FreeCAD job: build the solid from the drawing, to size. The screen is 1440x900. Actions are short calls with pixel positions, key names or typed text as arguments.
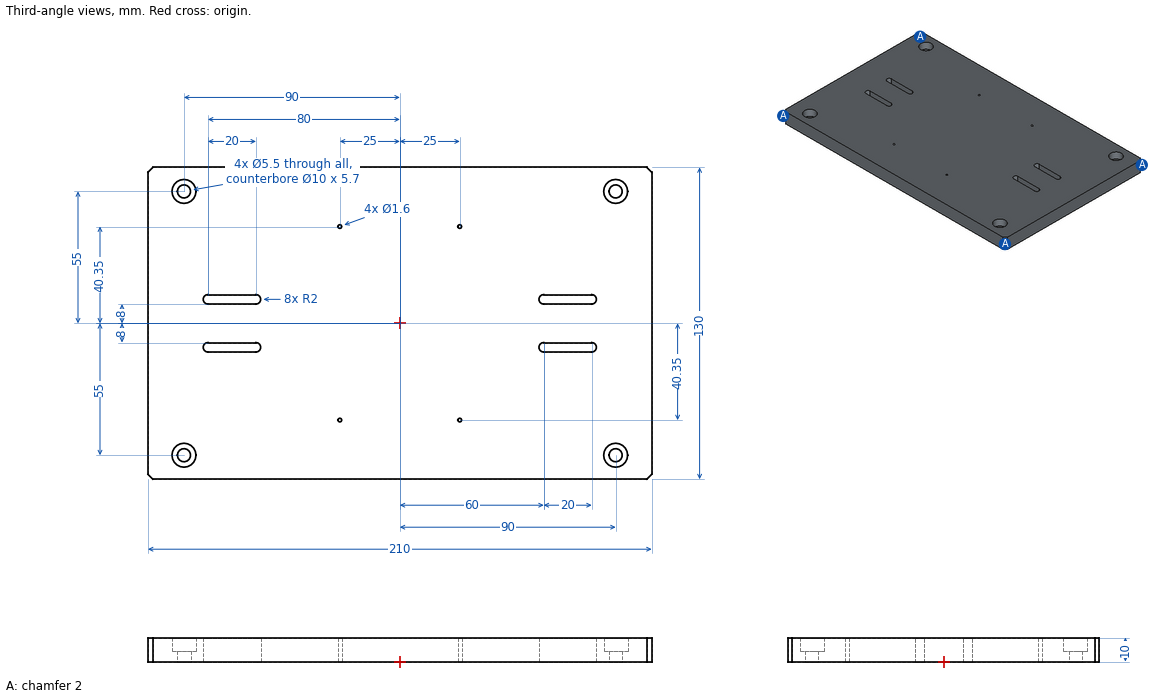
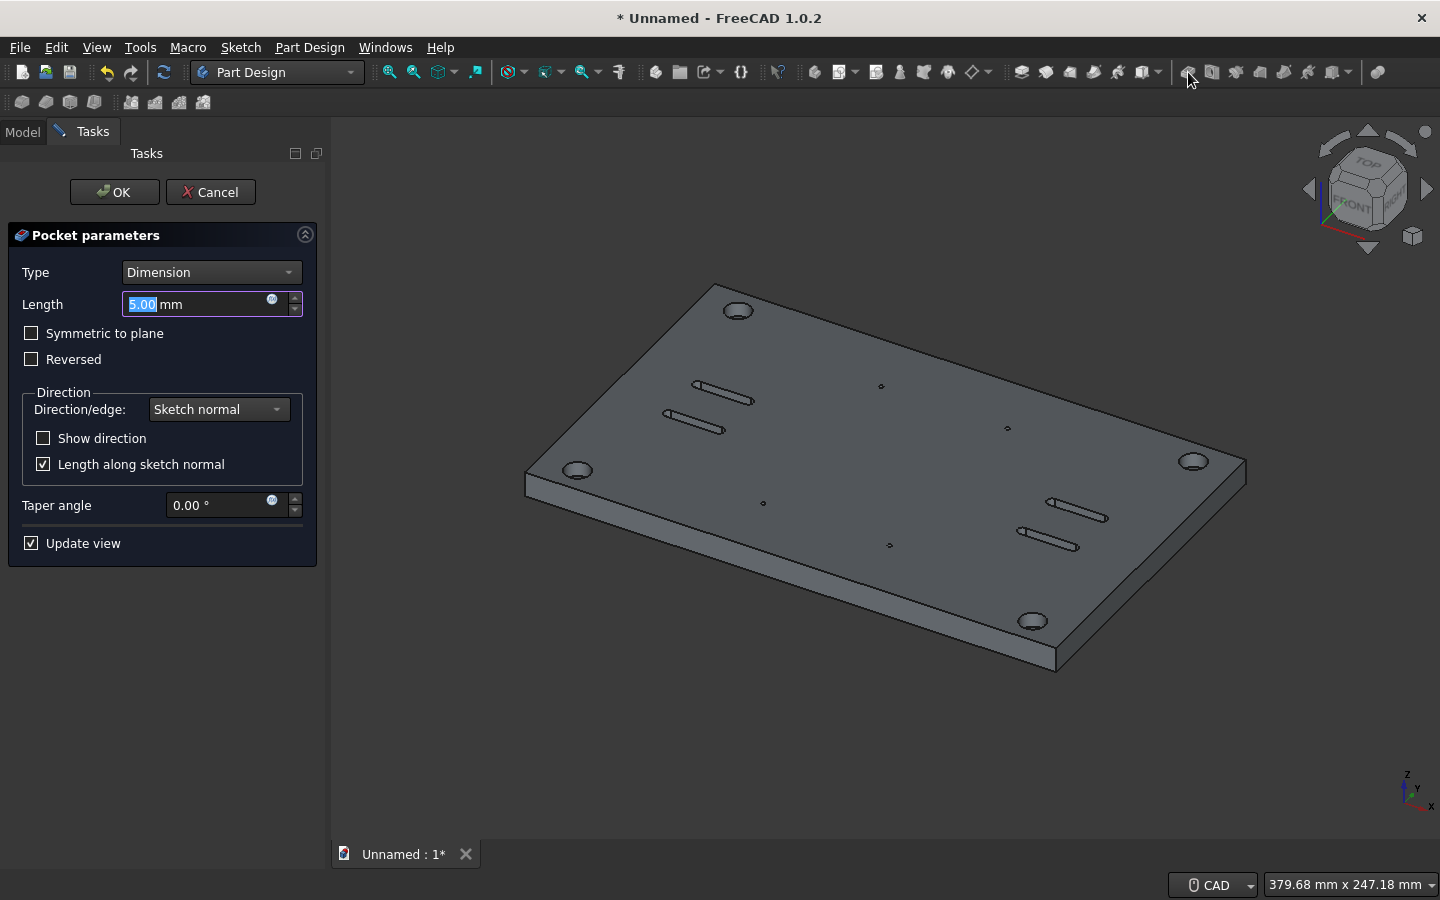
click(212, 272)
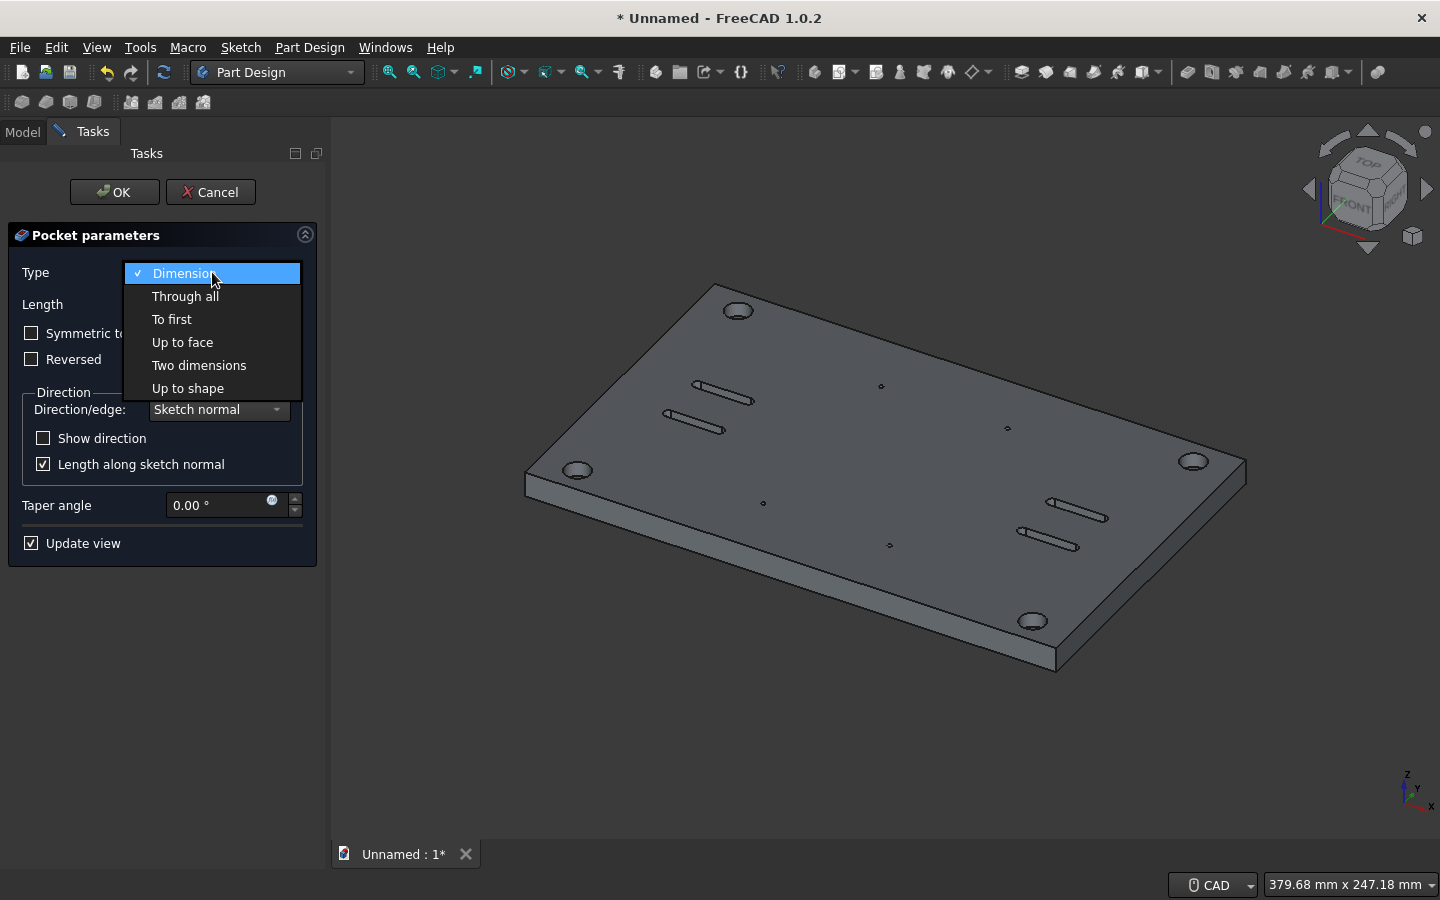
click(212, 296)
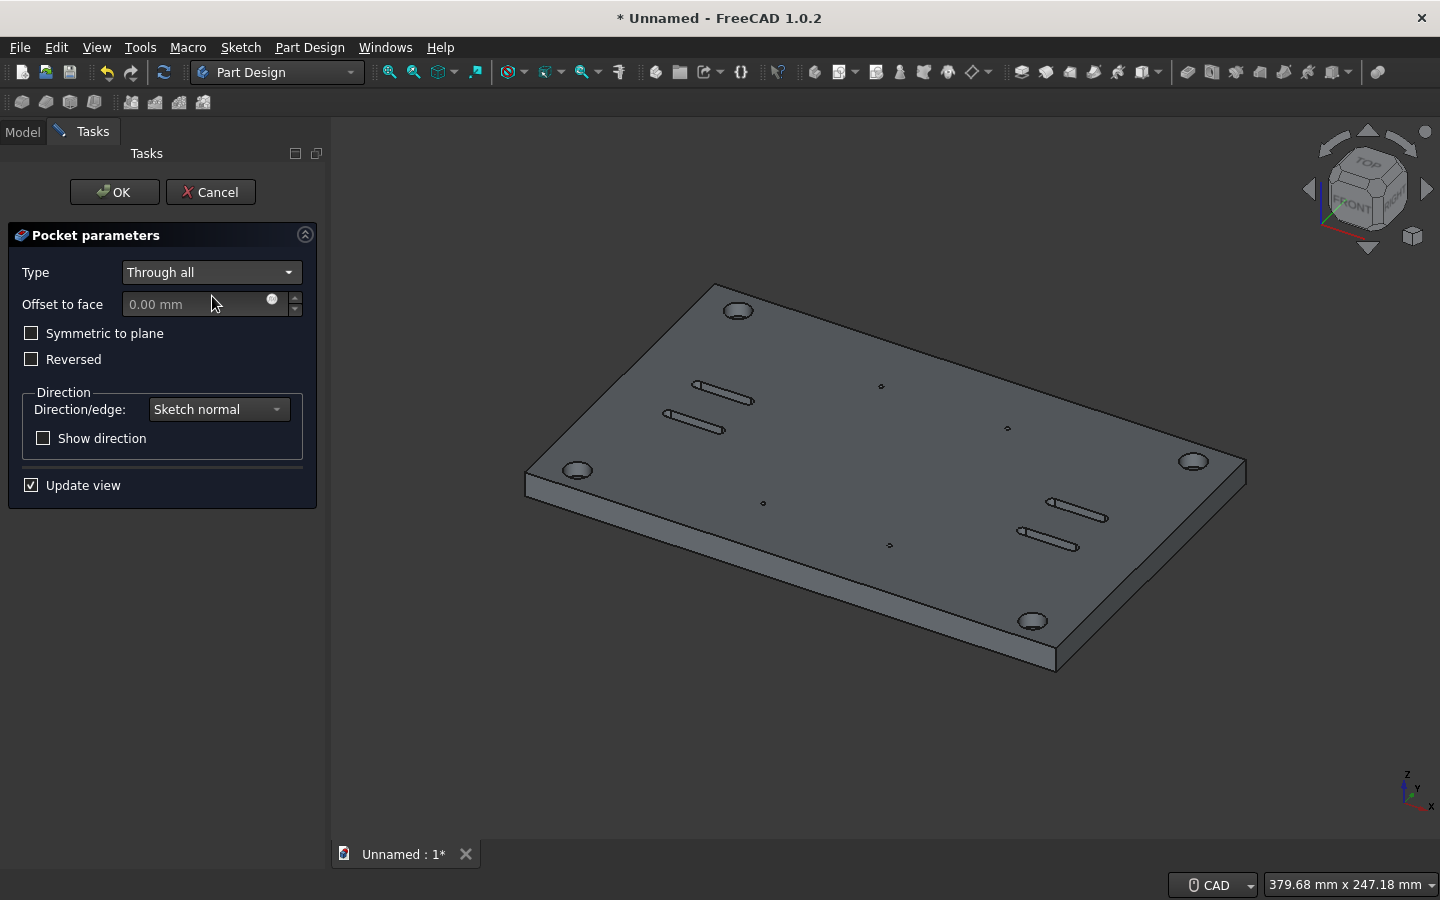
click(115, 192)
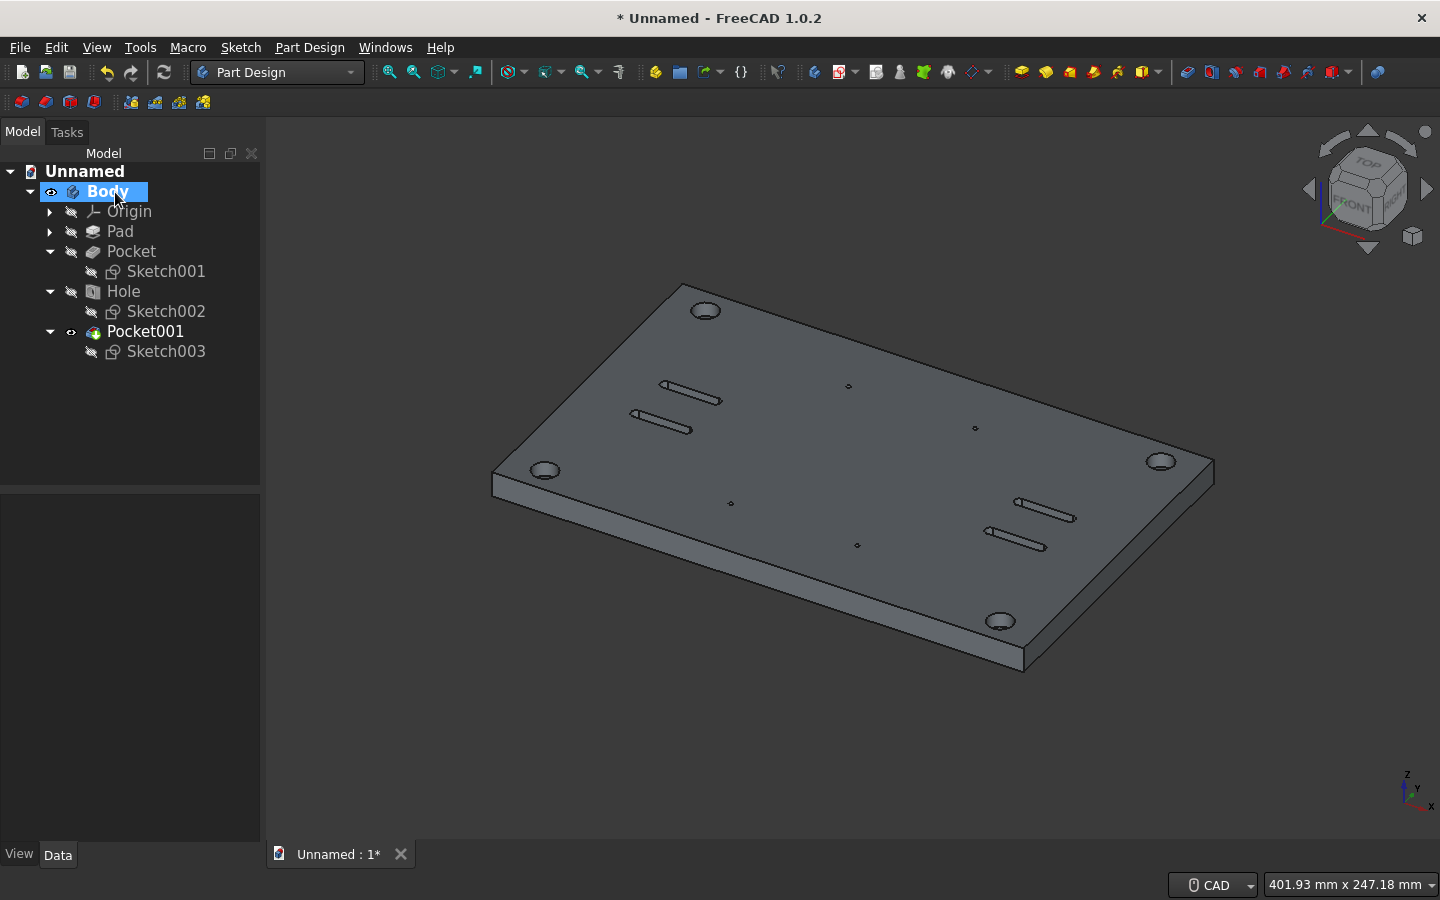
click(1024, 659)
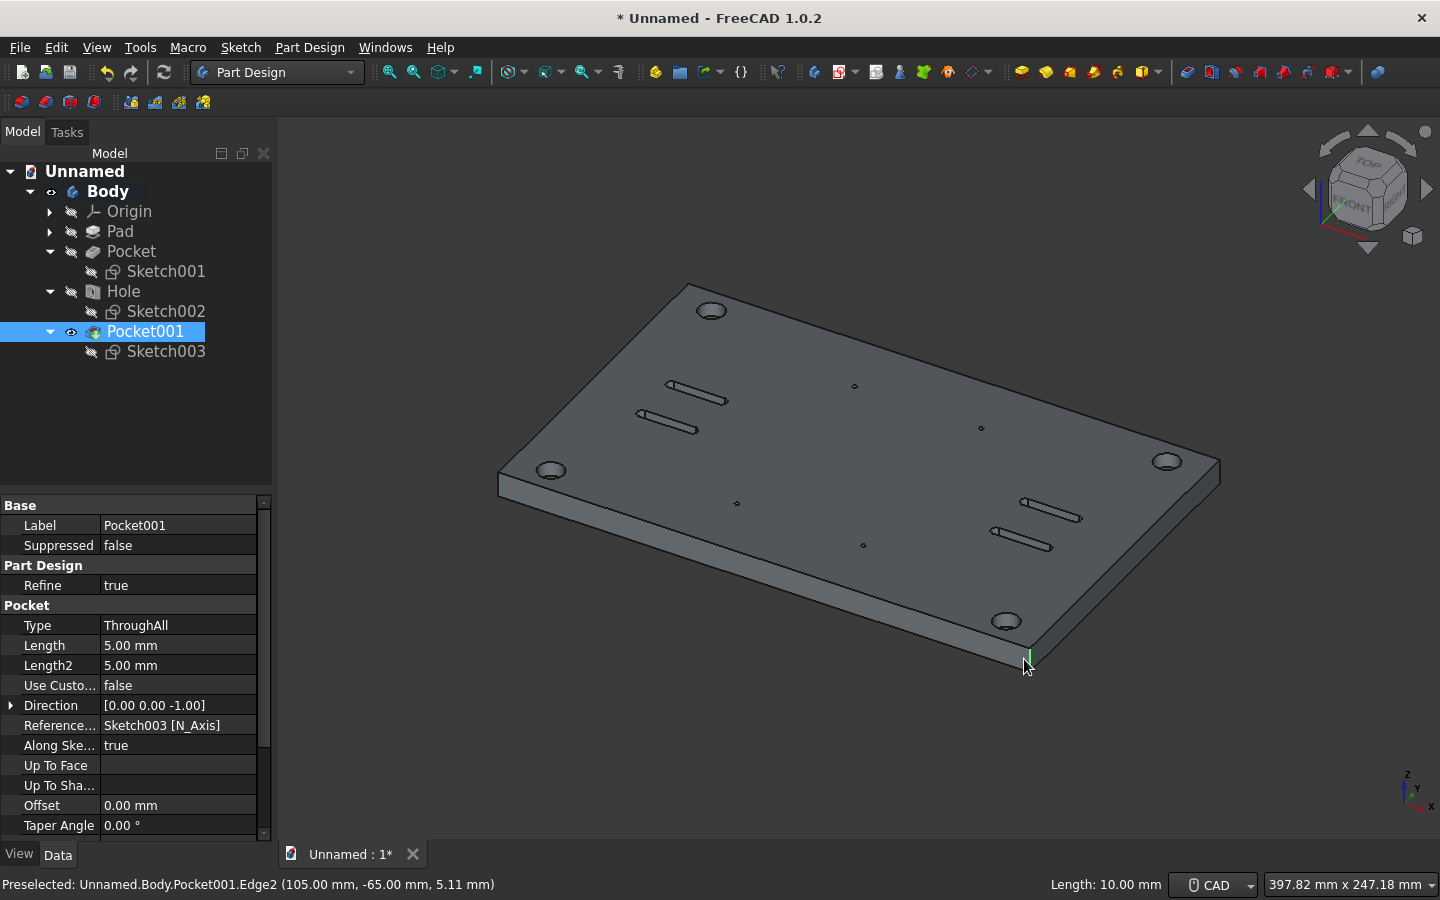
key(0)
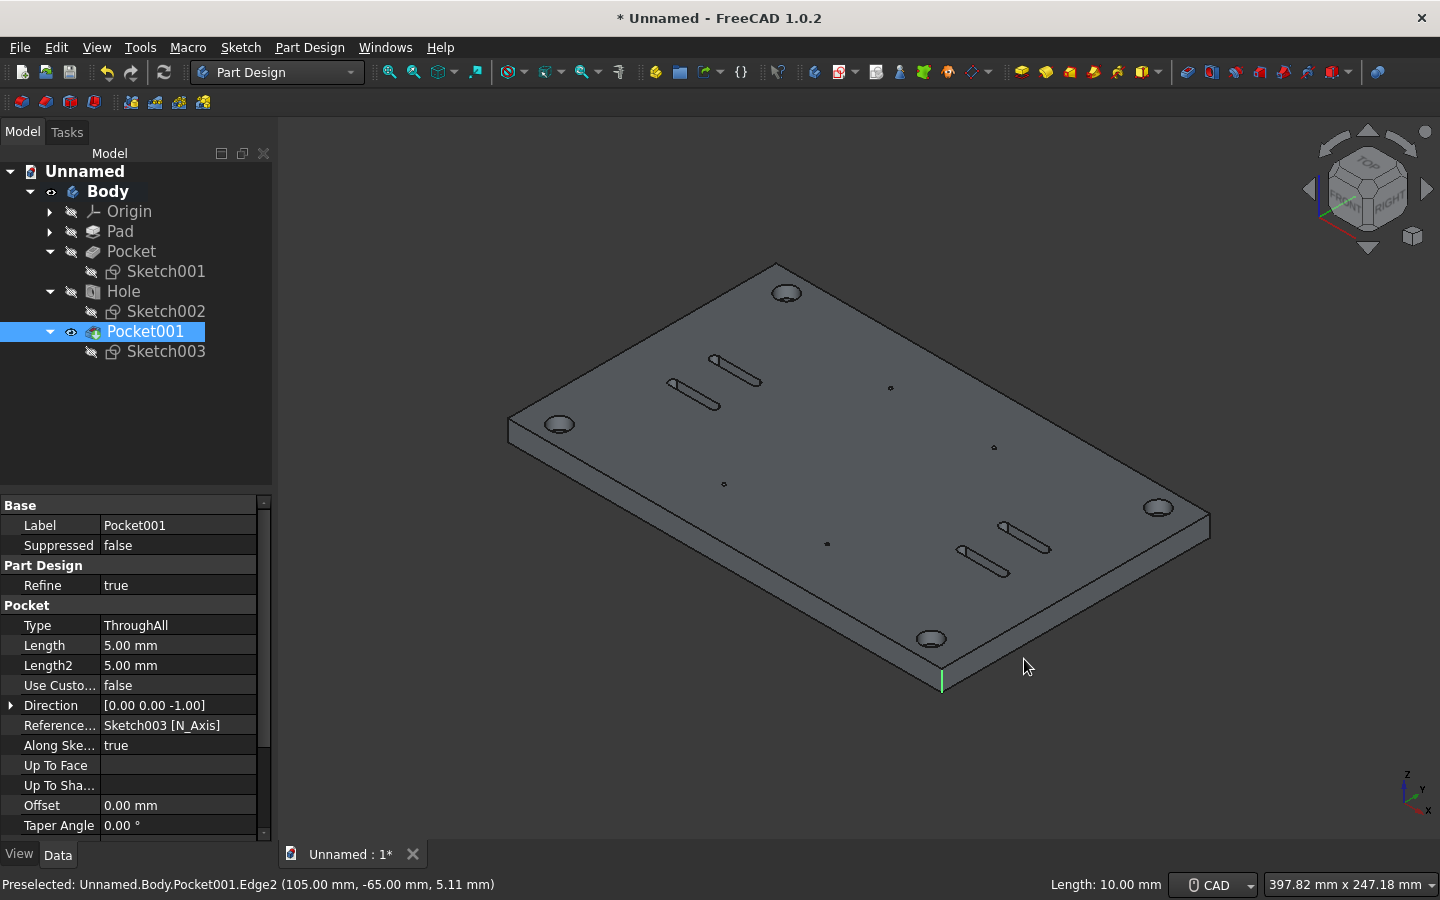
key(2)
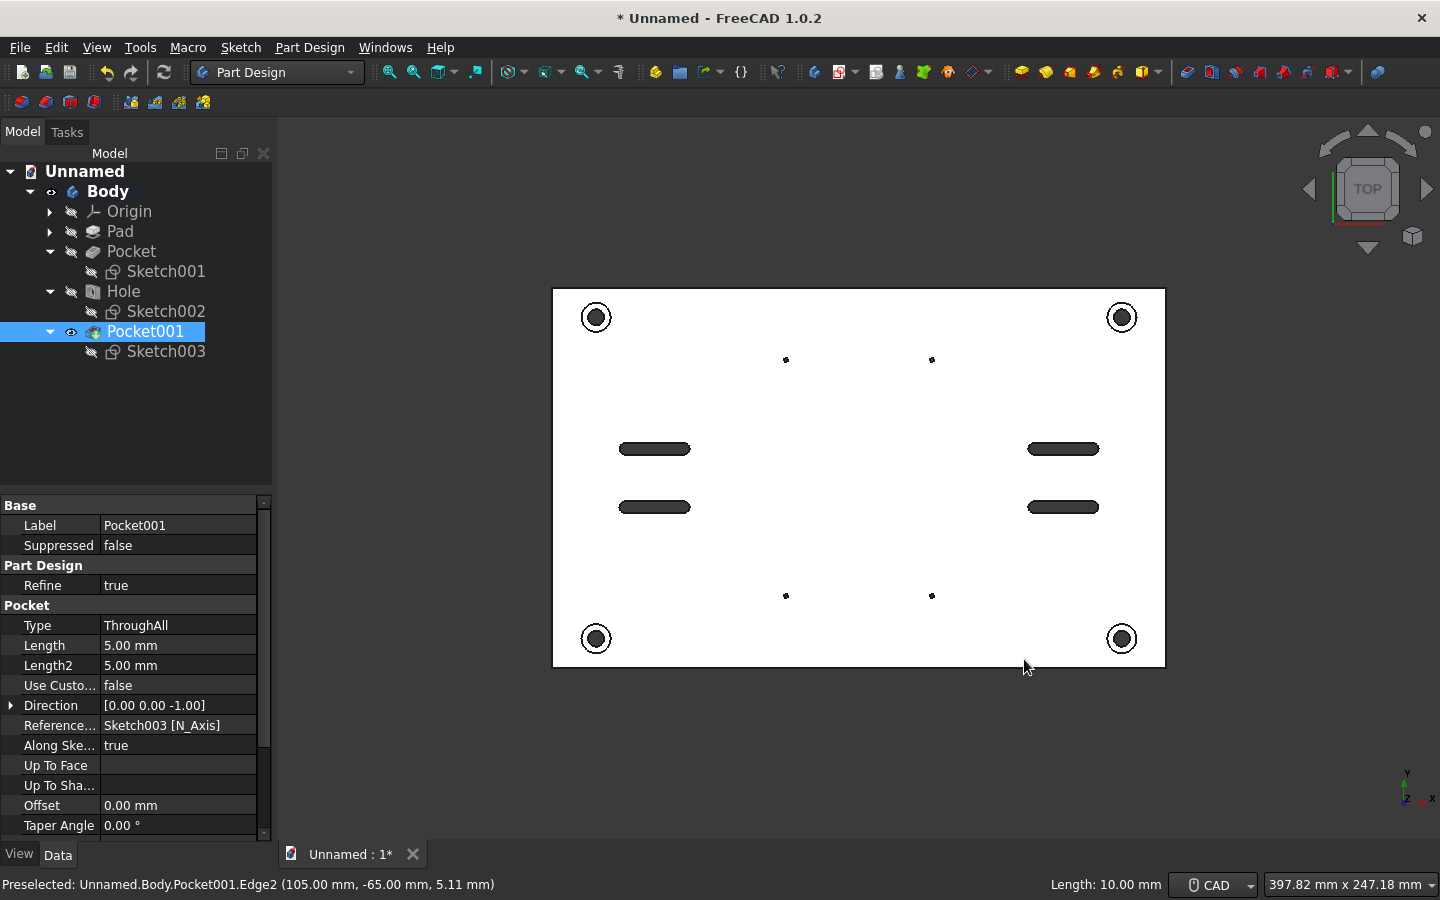
key(1)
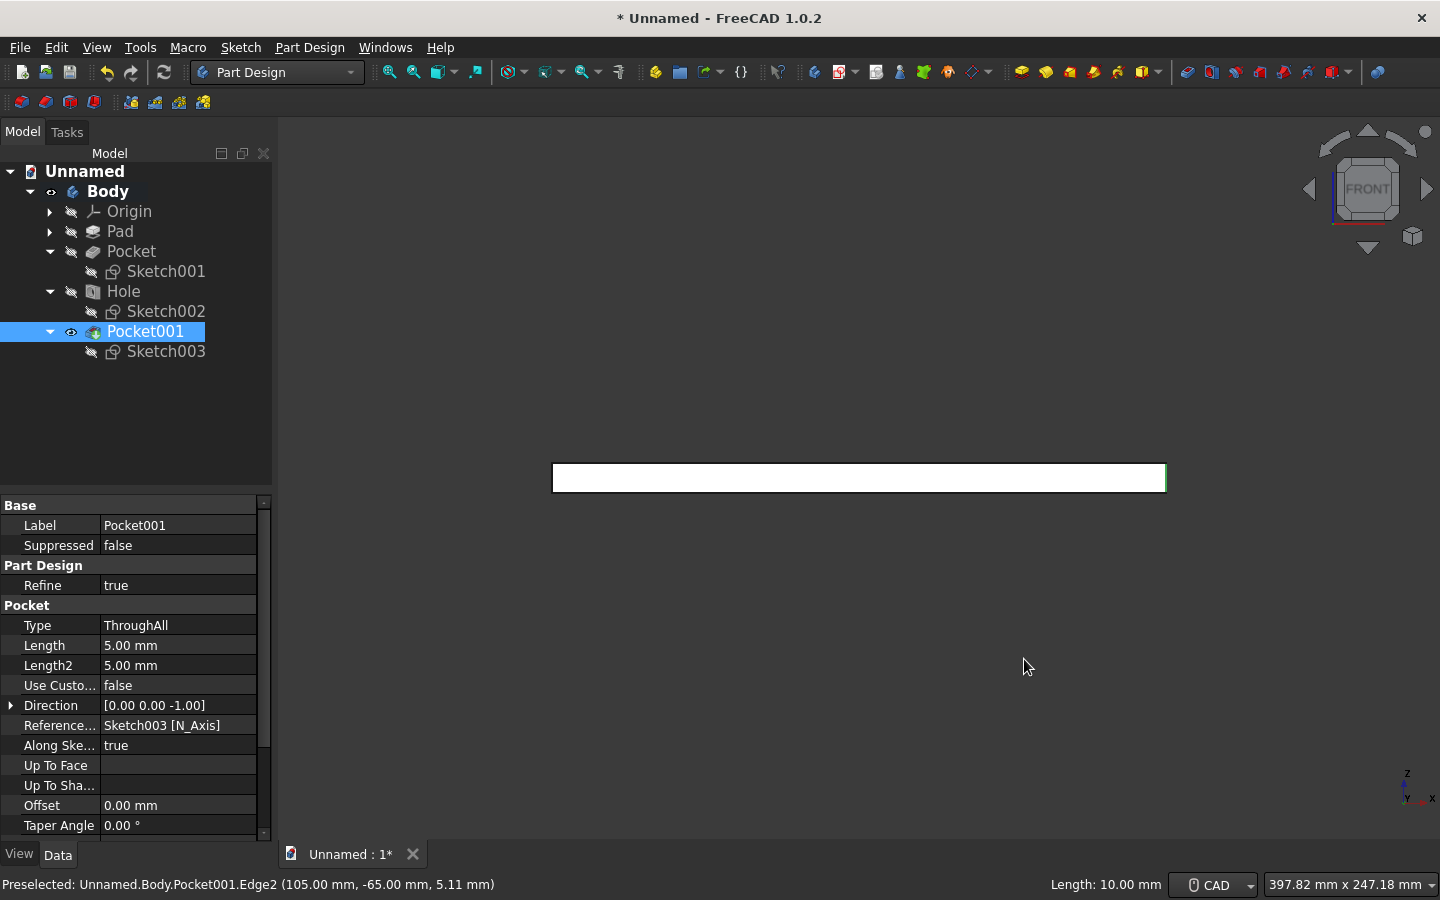
click(552, 477, ctrl)